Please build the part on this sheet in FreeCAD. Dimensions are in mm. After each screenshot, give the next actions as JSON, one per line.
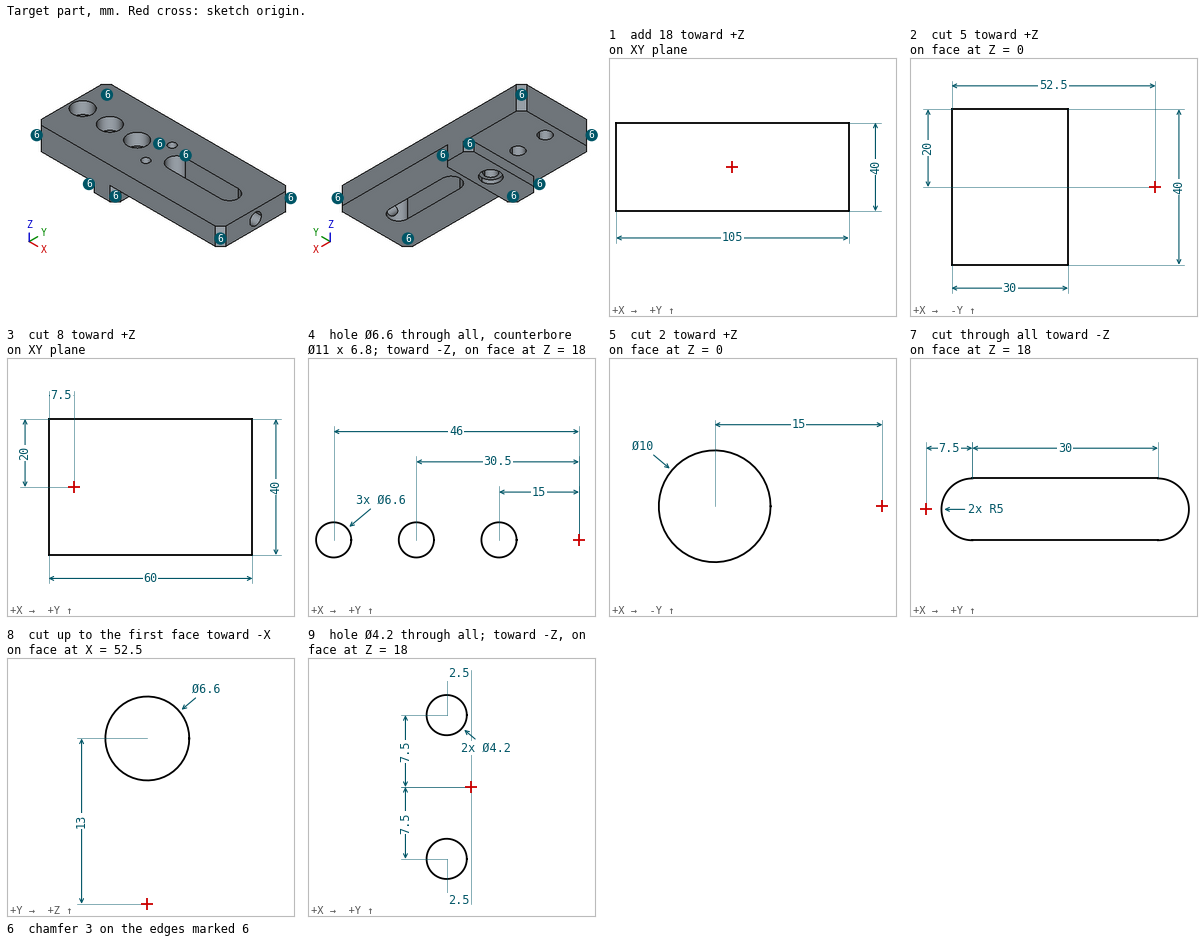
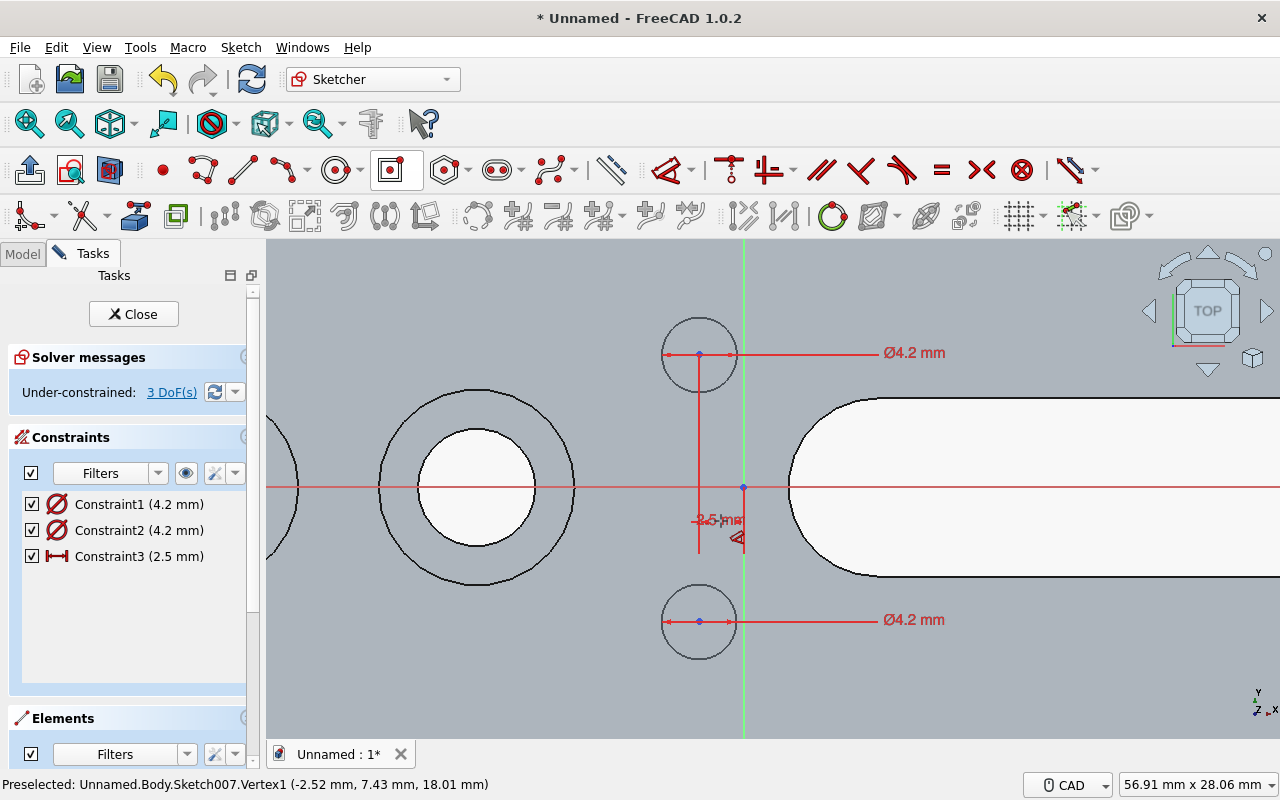
{"action": "left_click", "coordinate": [699, 355]}
{"action": "left_click", "coordinate": [778, 421]}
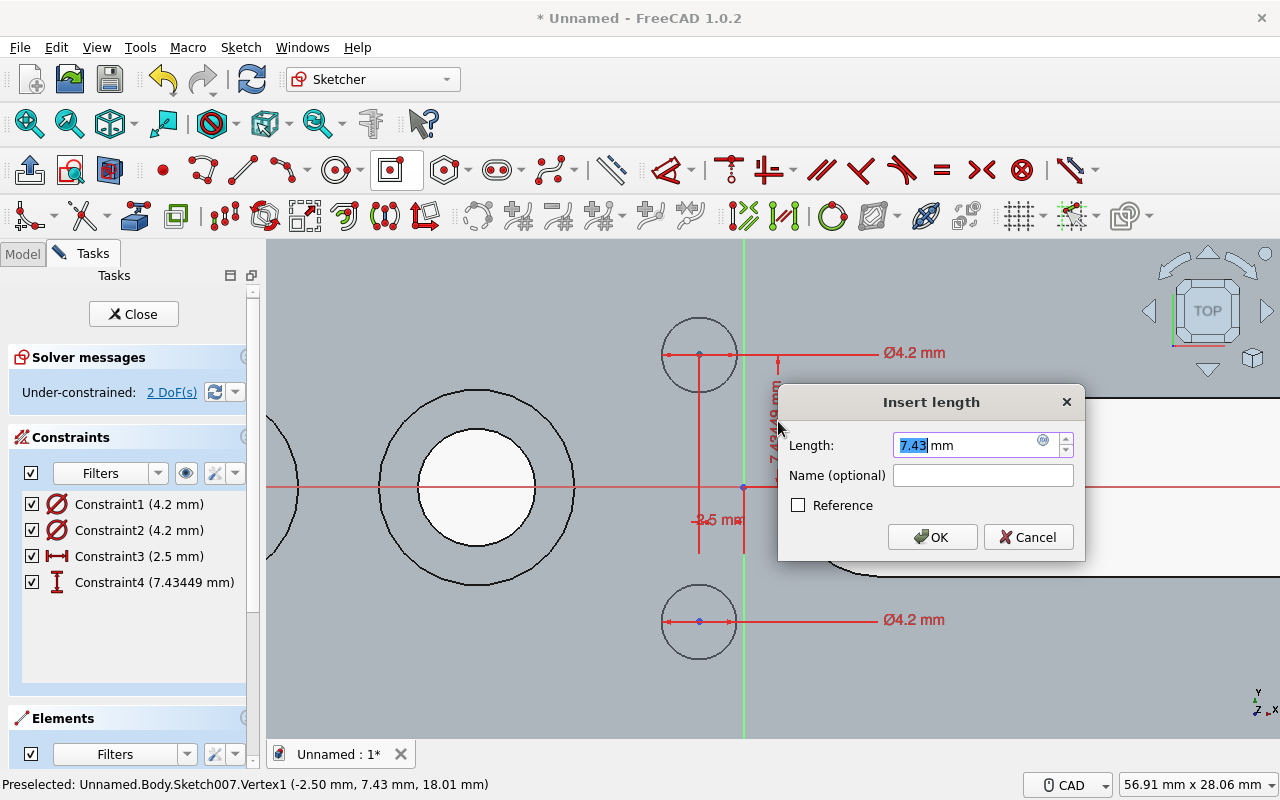
{"action": "type", "text": "7.5"}
{"action": "key", "text": "Return"}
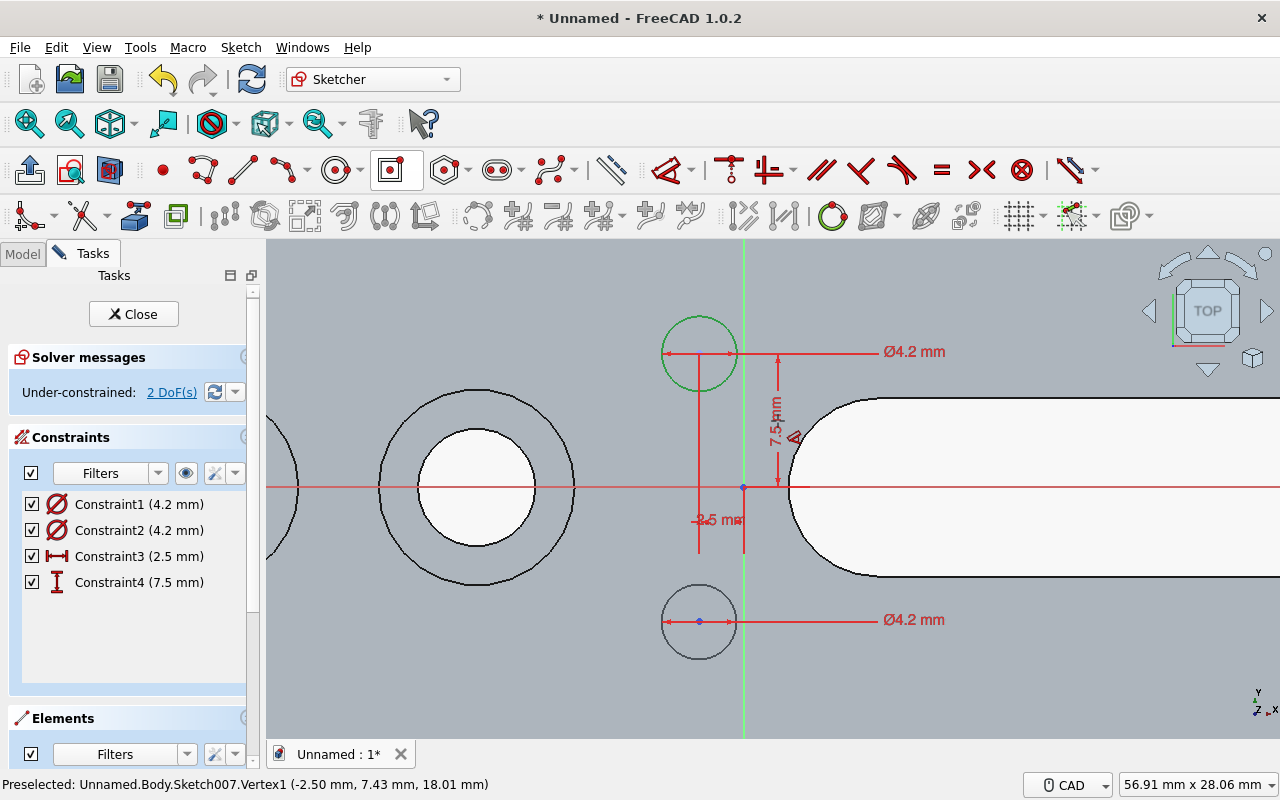
{"action": "left_click", "coordinate": [699, 622]}
{"action": "left_click", "coordinate": [721, 453]}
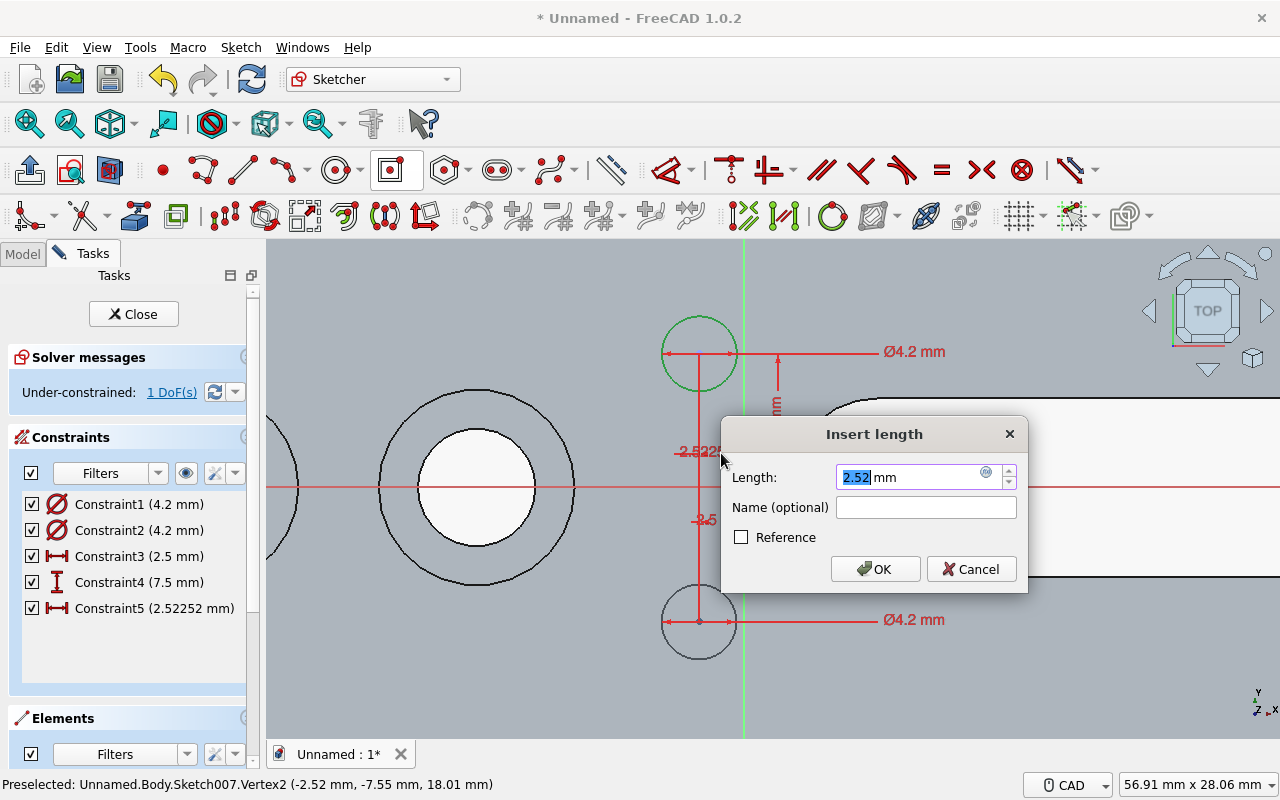
{"action": "type", "text": "2.5"}
{"action": "key", "text": "Return"}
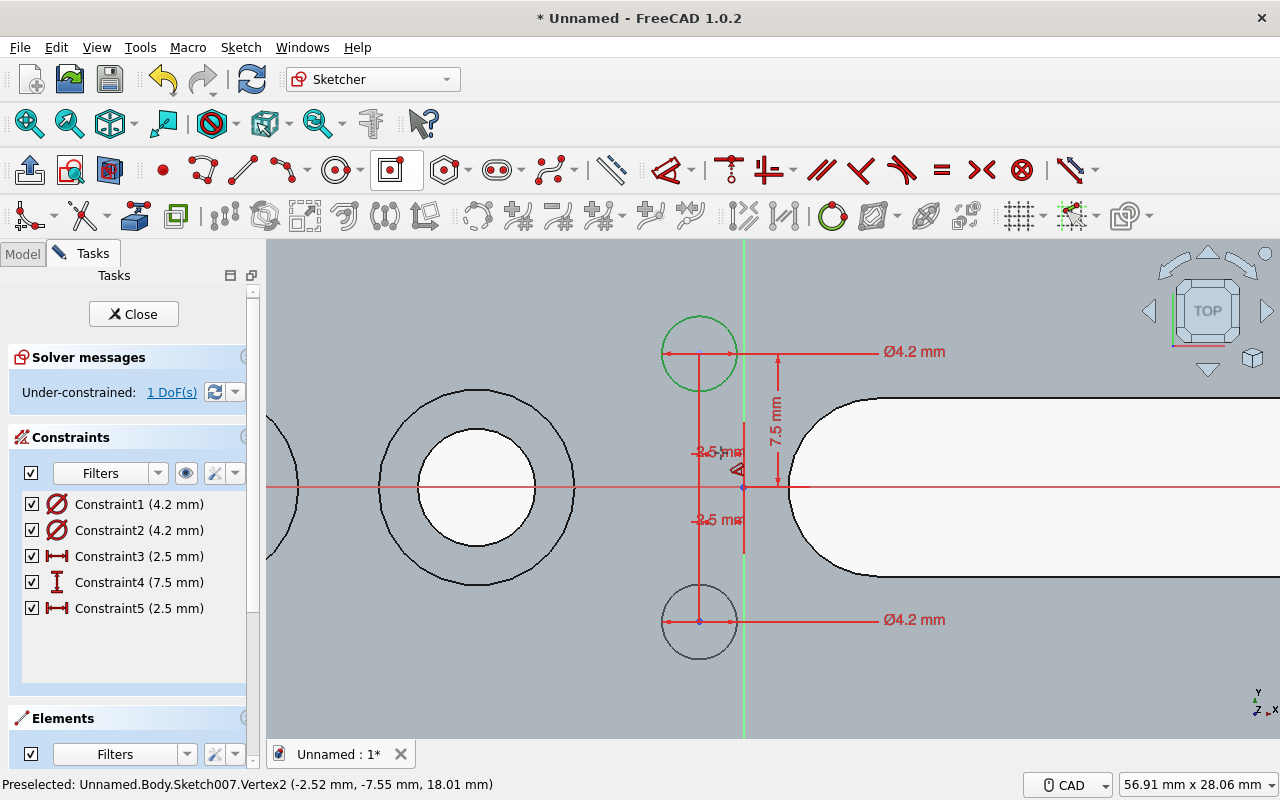
{"action": "left_click", "coordinate": [699, 622]}
{"action": "left_click", "coordinate": [778, 555]}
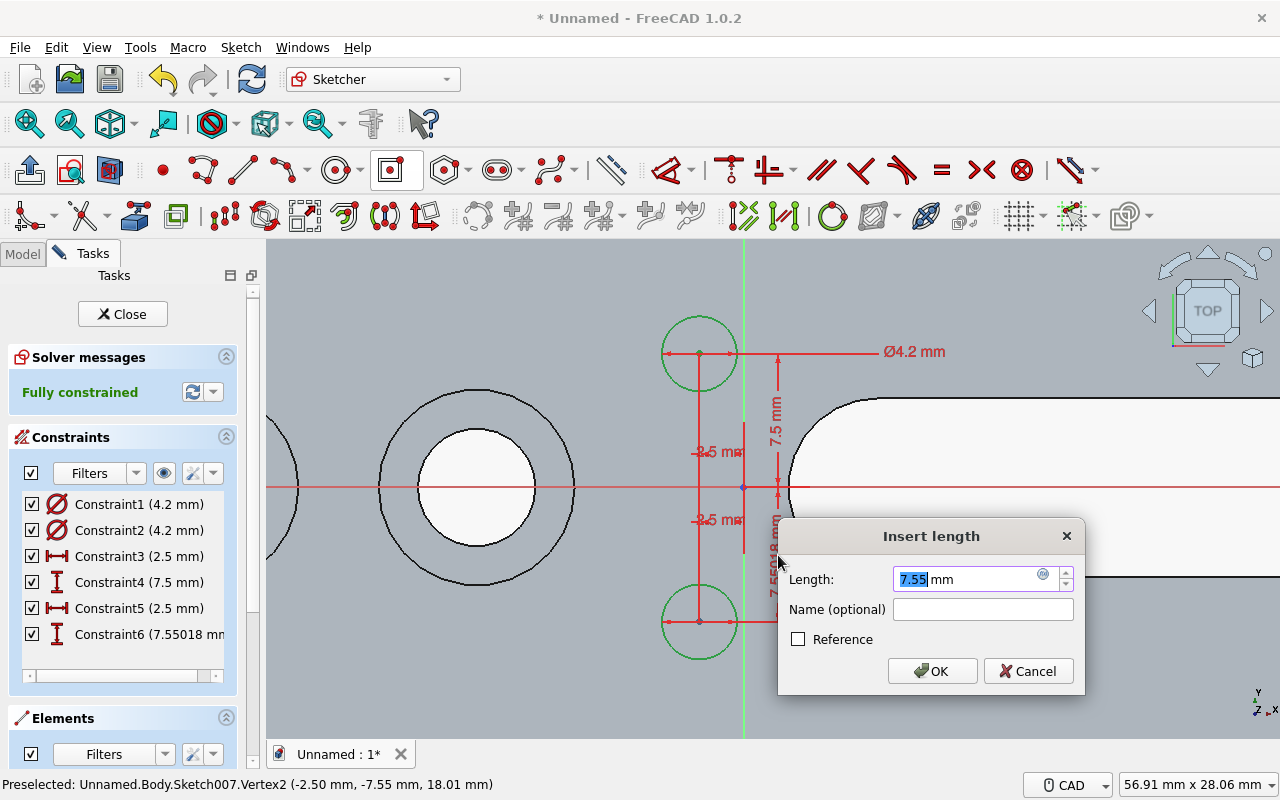
{"action": "type", "text": "7.5"}
{"action": "key", "text": "Return"}
{"action": "key", "text": "Escape"}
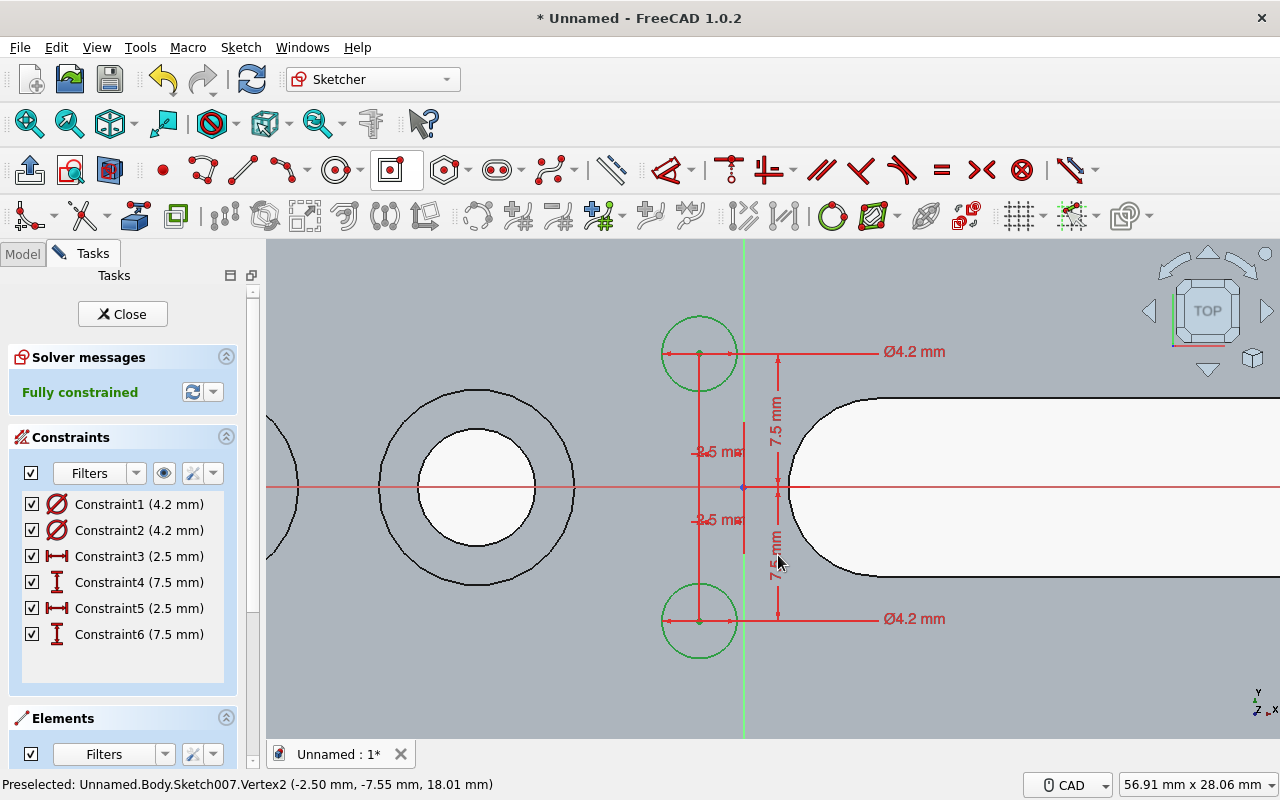
{"action": "left_click", "coordinate": [123, 314]}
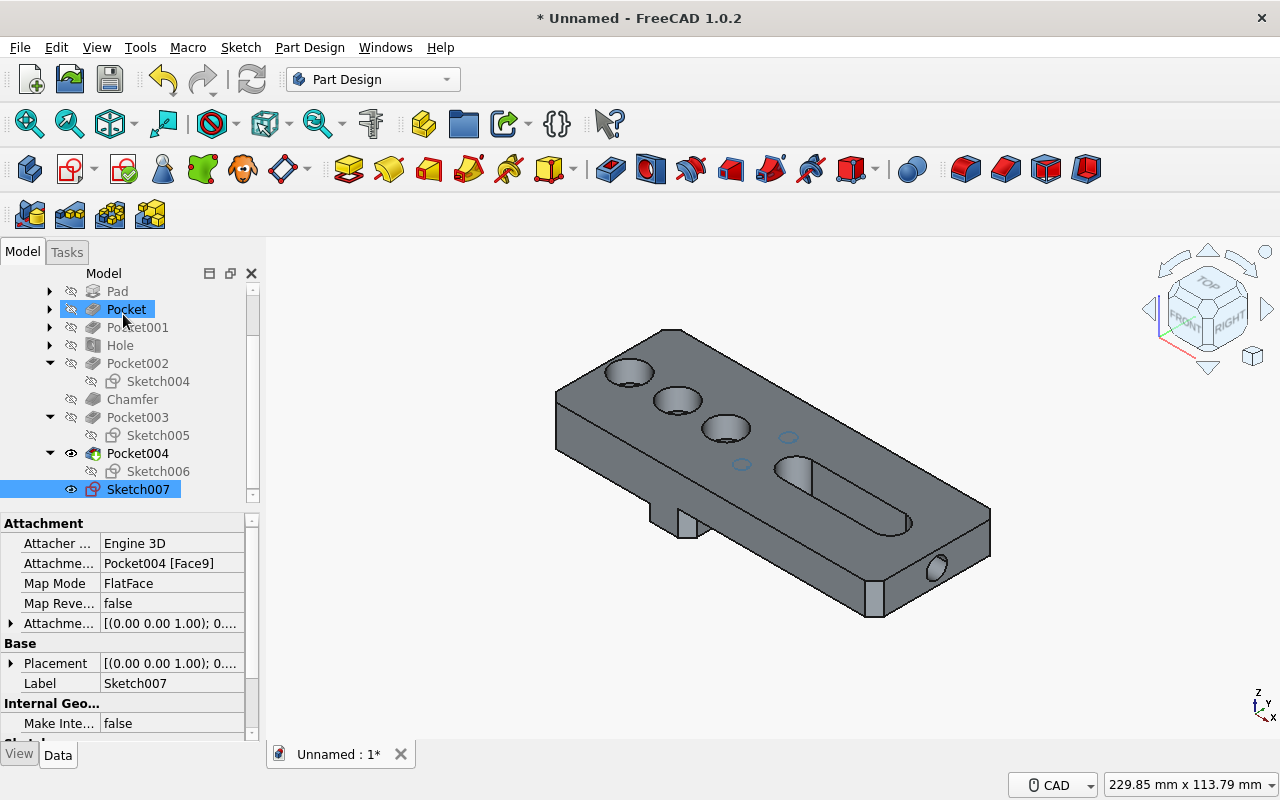
{"action": "left_click", "coordinate": [652, 170]}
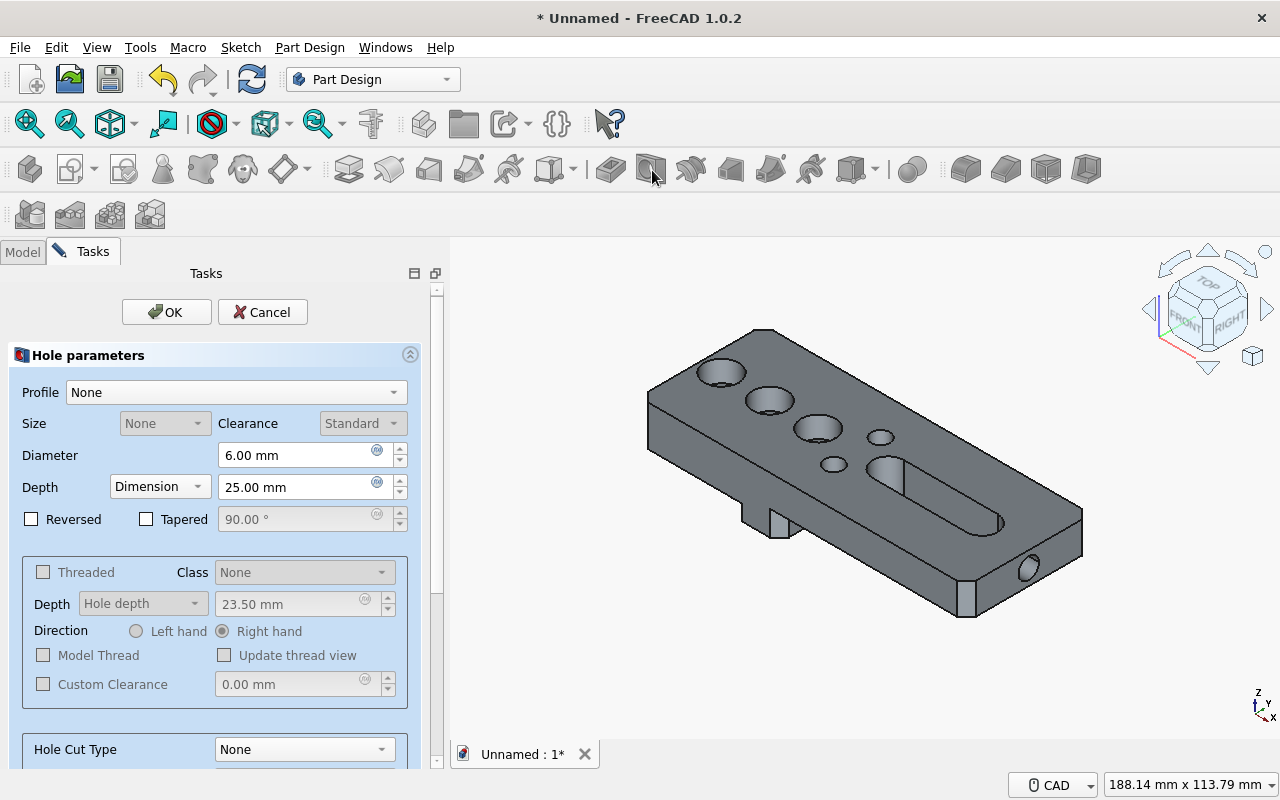
{"action": "triple_click", "coordinate": [305, 455]}